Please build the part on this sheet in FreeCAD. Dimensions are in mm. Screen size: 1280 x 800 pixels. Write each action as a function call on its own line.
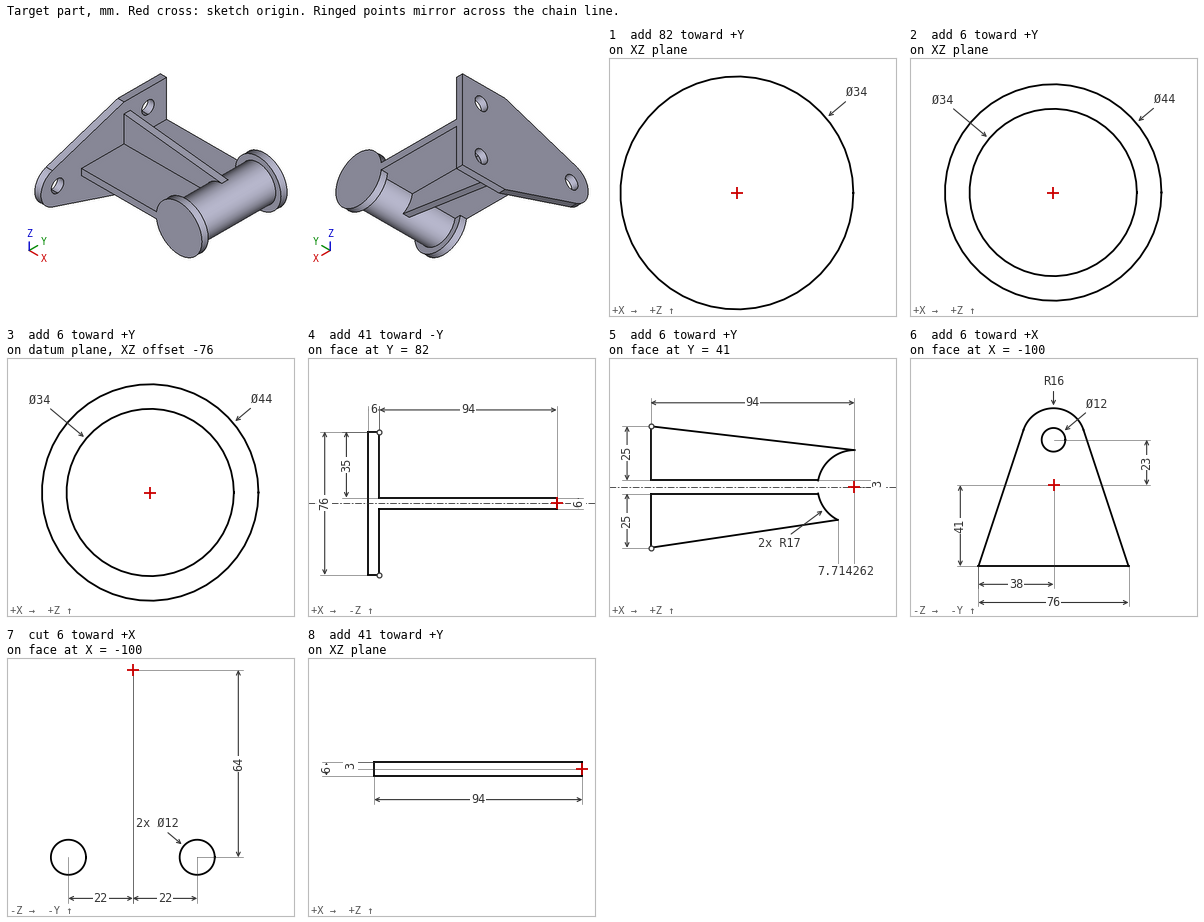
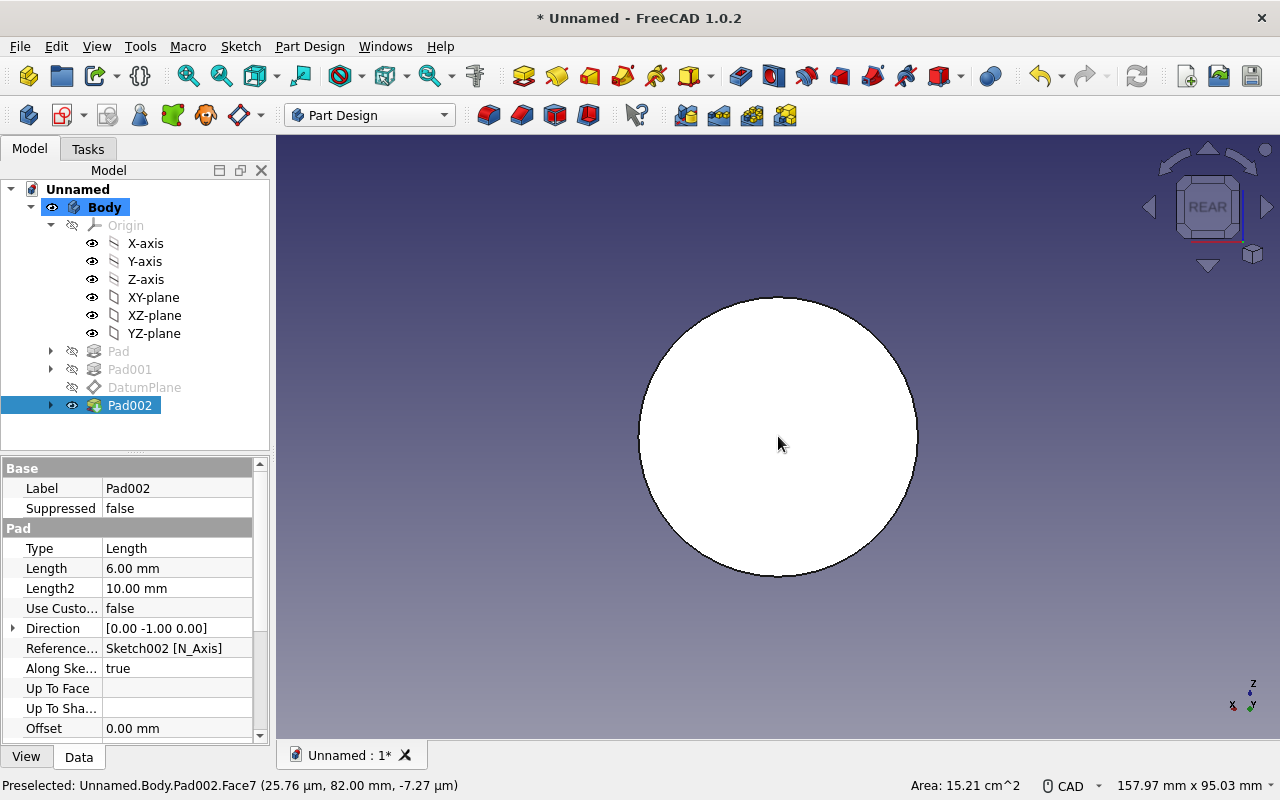
click(62, 116)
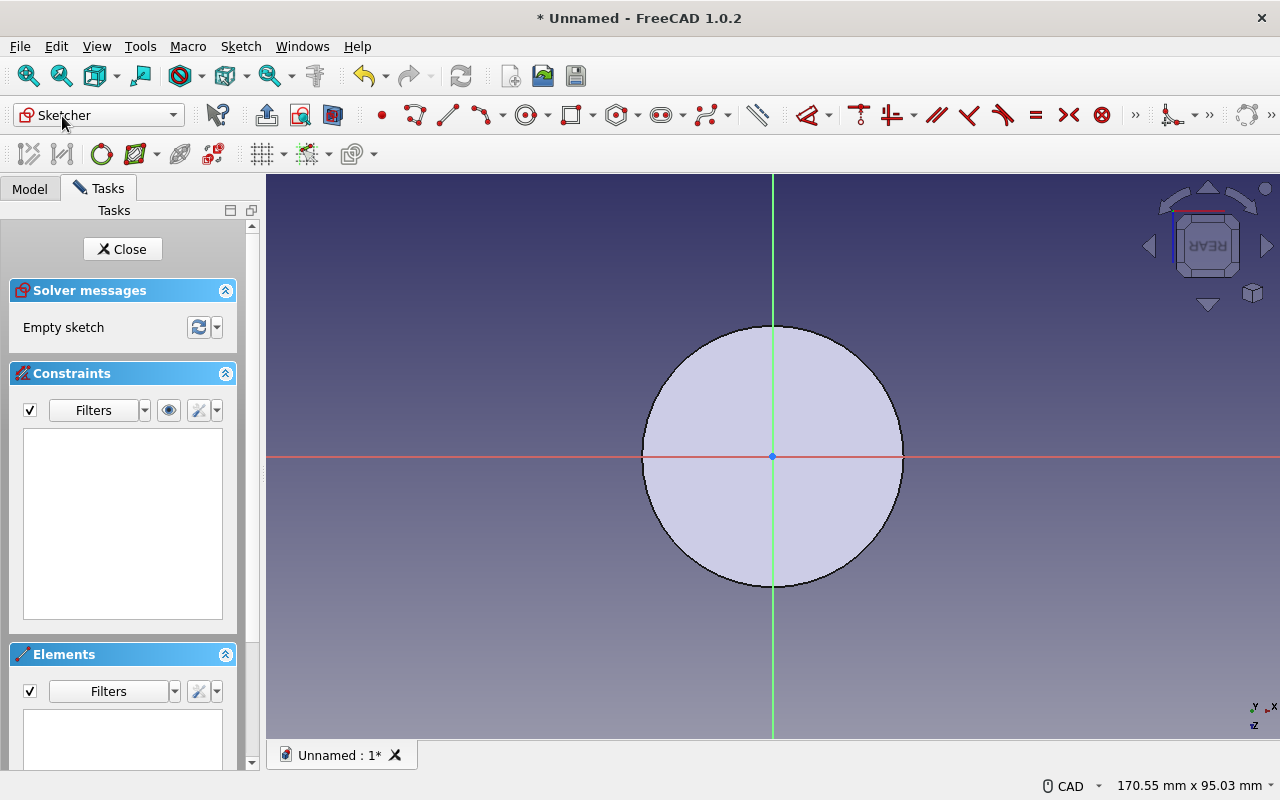
scroll(1115, 456, down, 1)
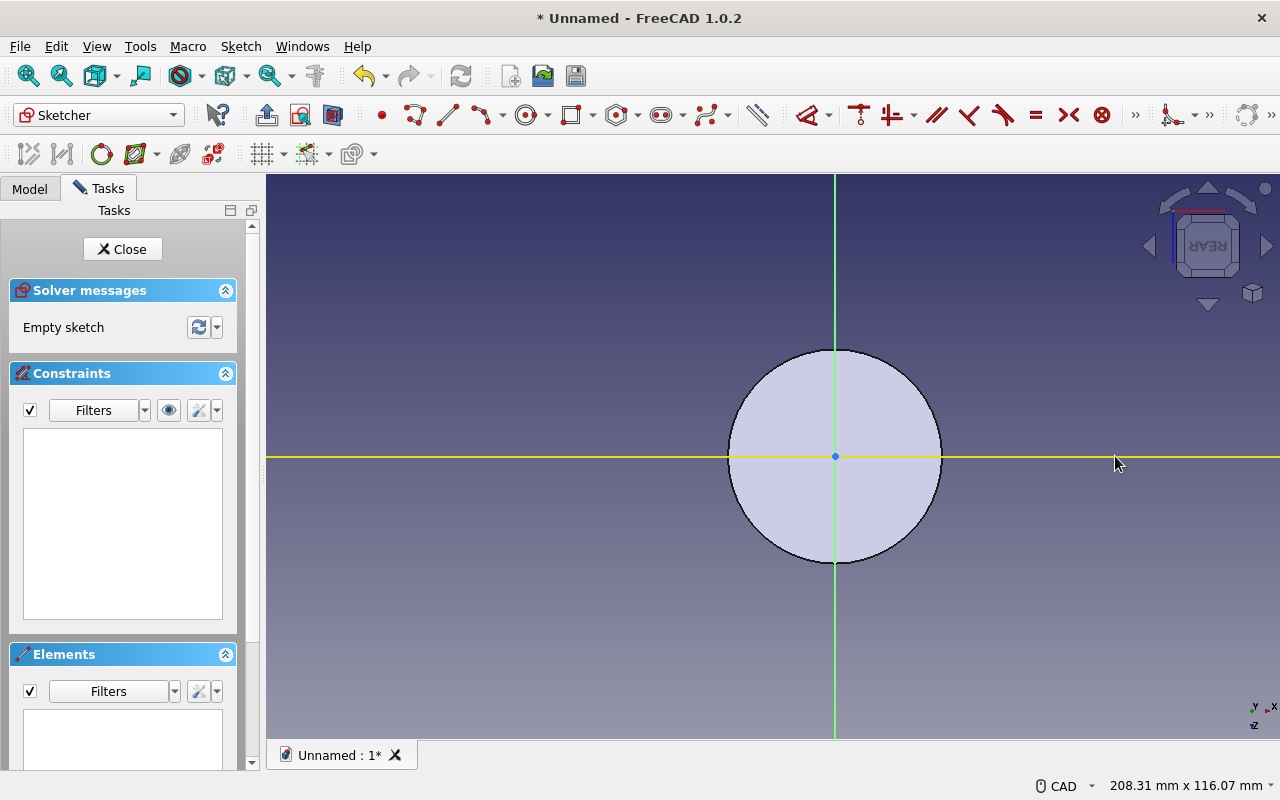
key(g)
key(m)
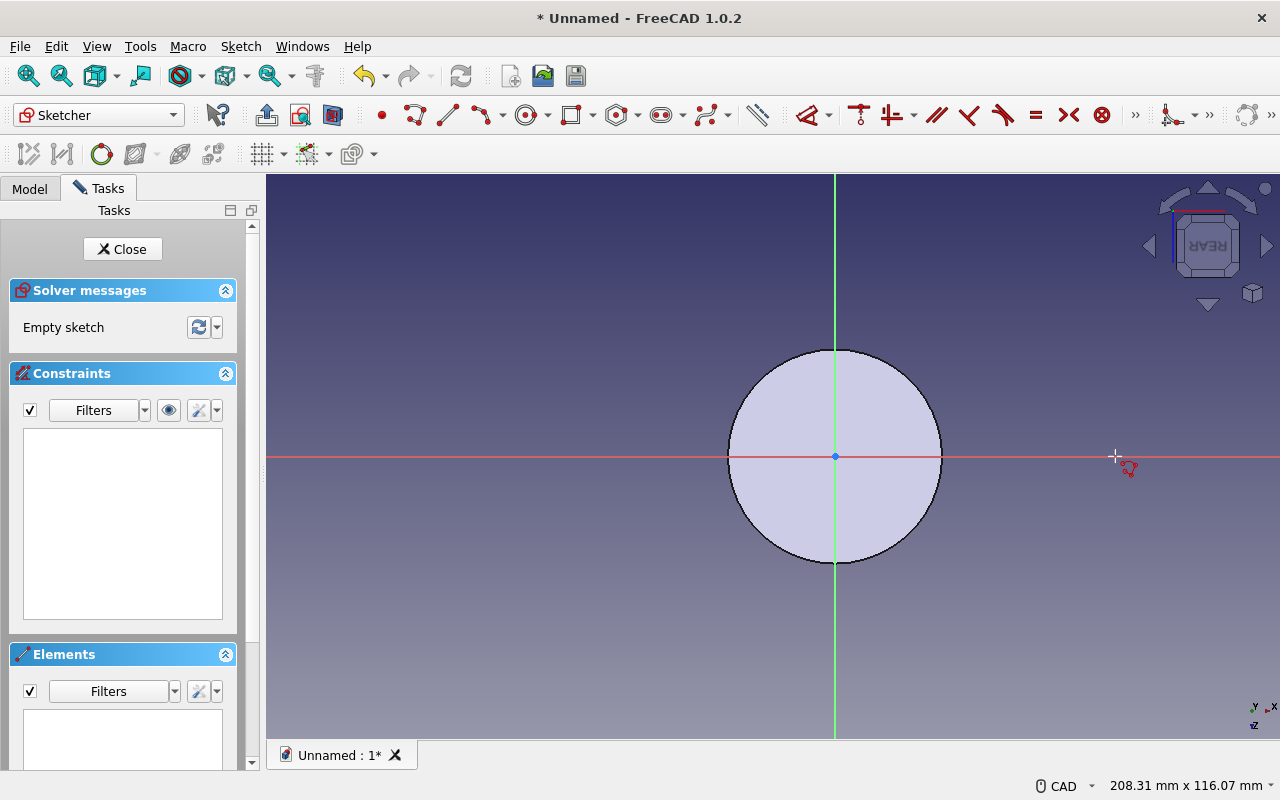
click(835, 471)
click(826, 442)
click(377, 442)
click(377, 272)
click(348, 272)
click(348, 642)
click(377, 642)
click(377, 471)
click(835, 472)
key(Escape)
key(Escape)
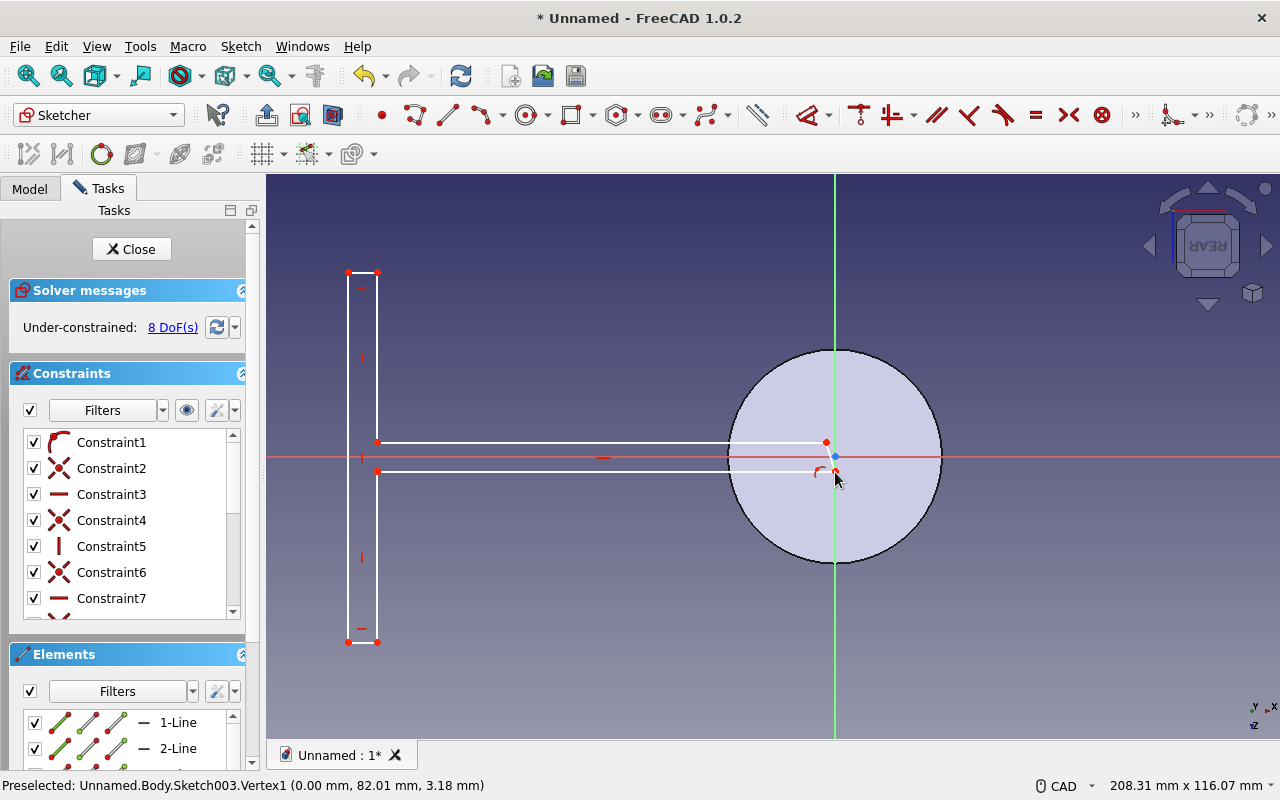
click(831, 460)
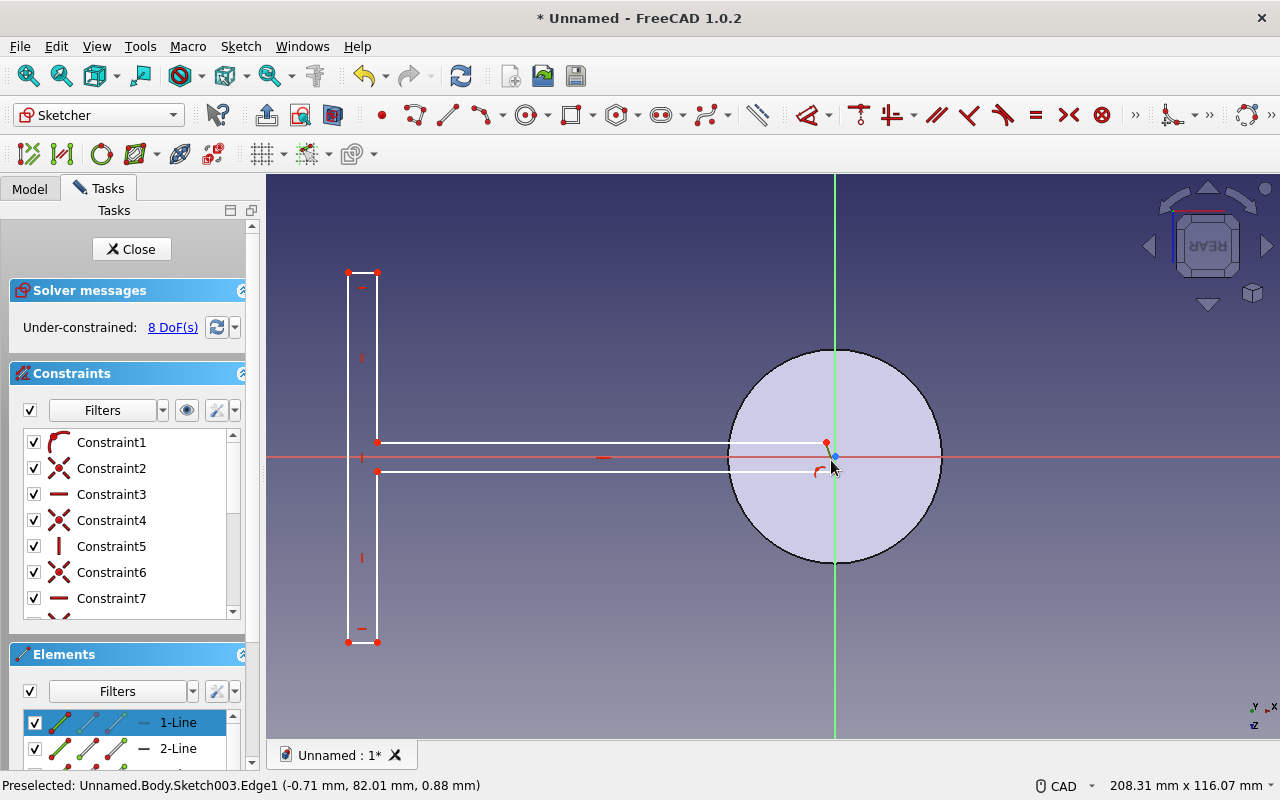
key(v)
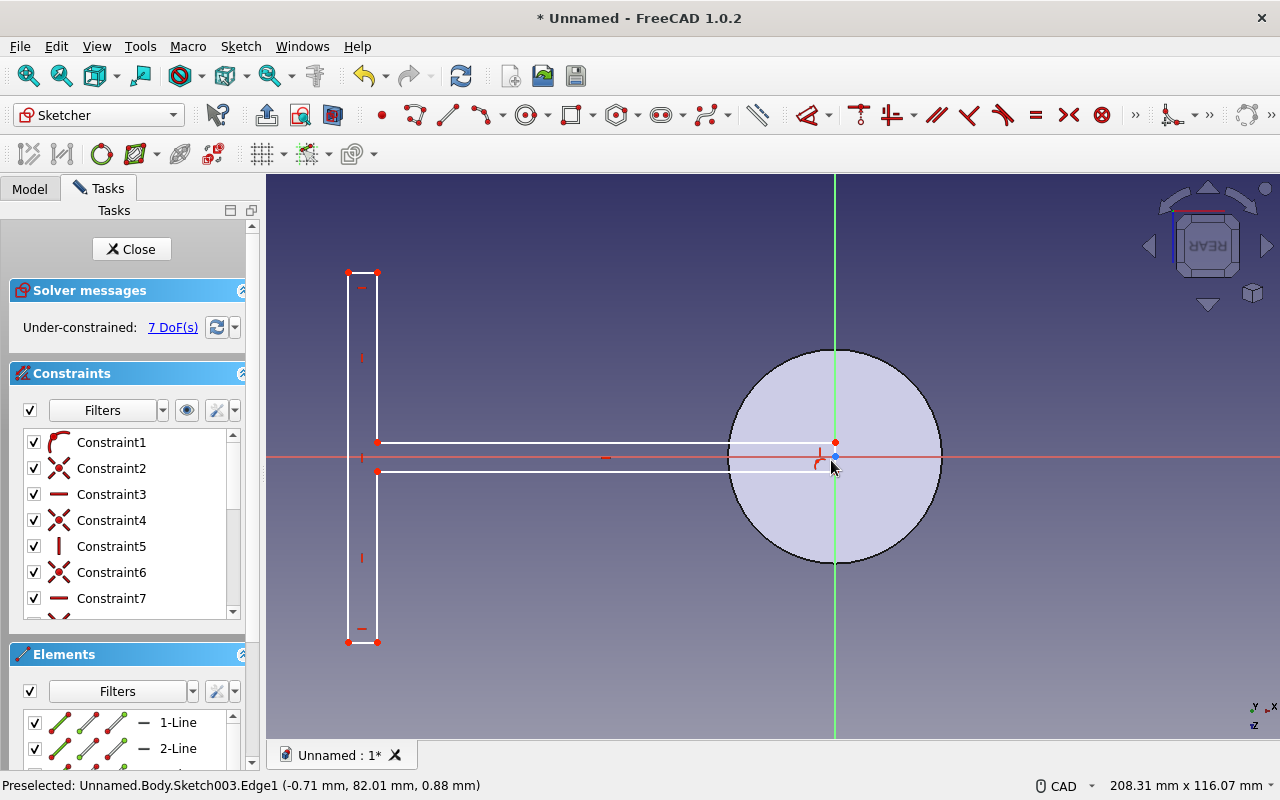
click(377, 273)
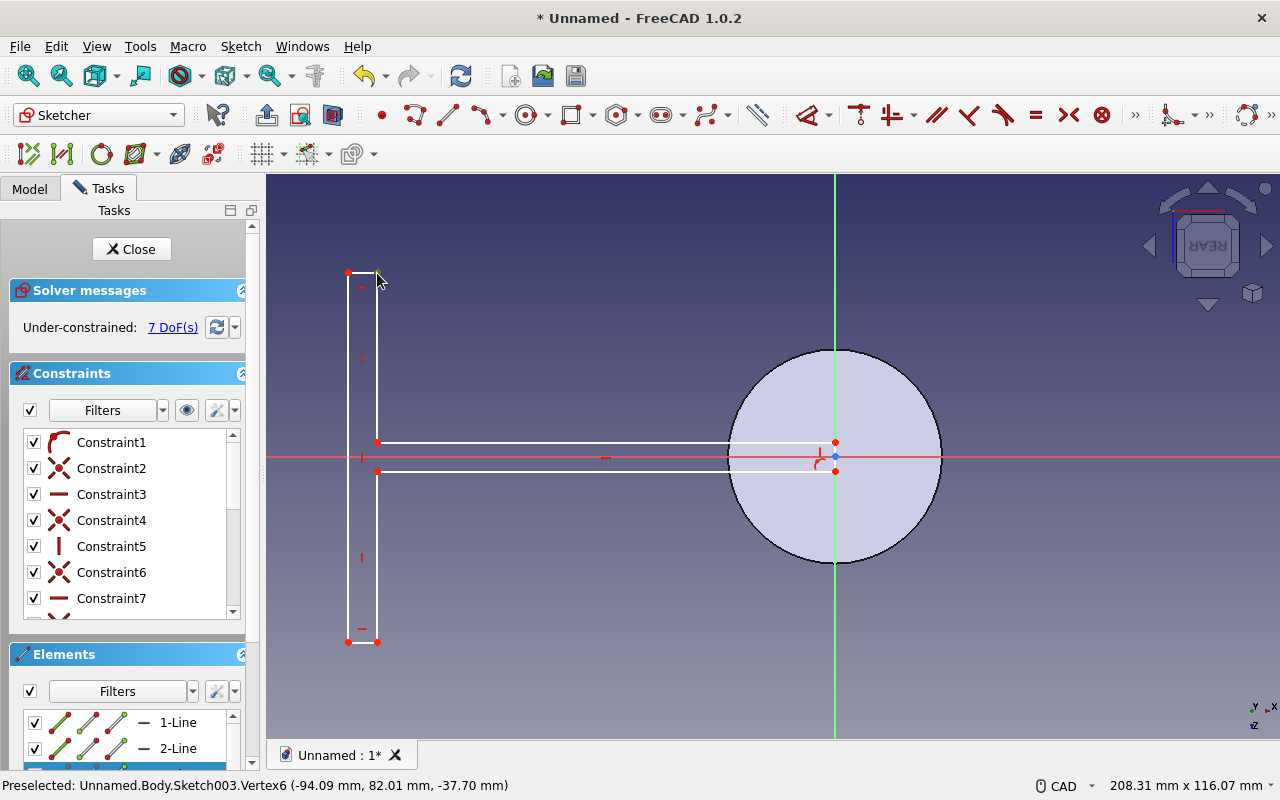
click(377, 643)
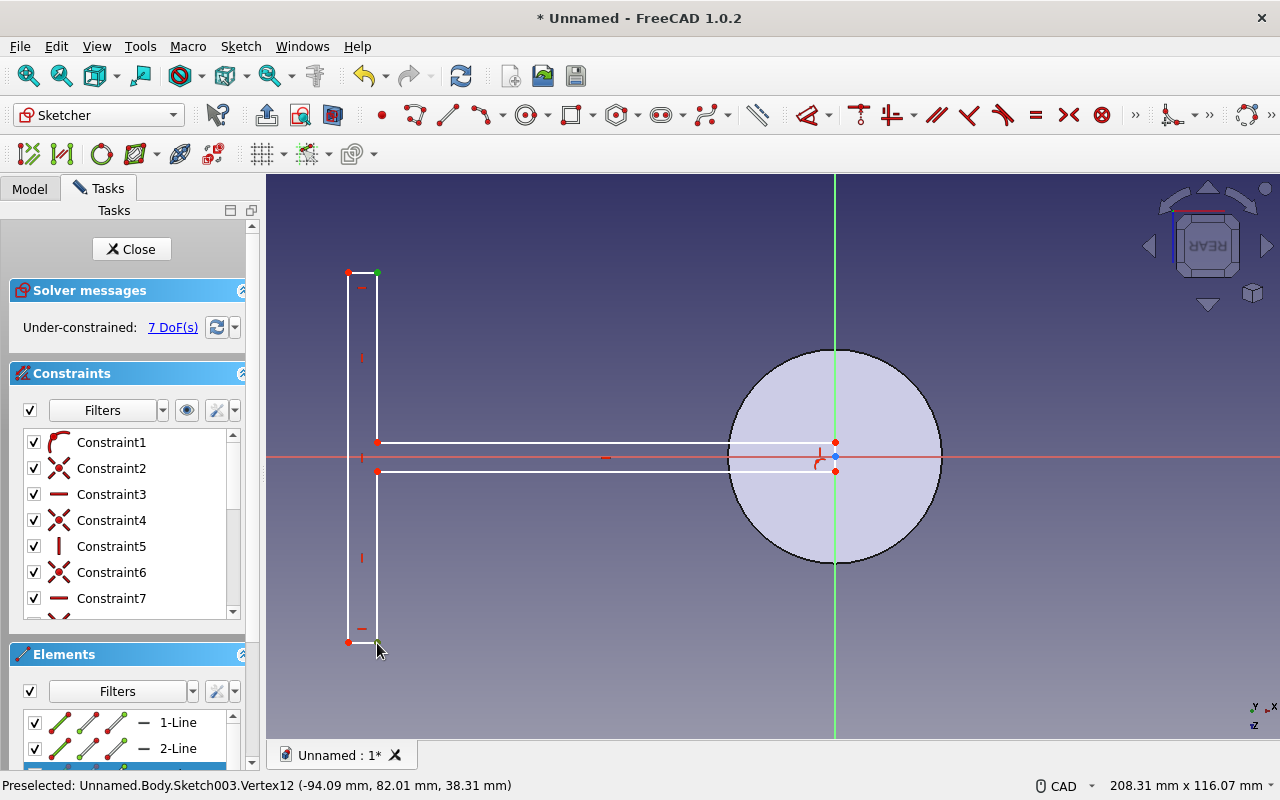
click(880, 457)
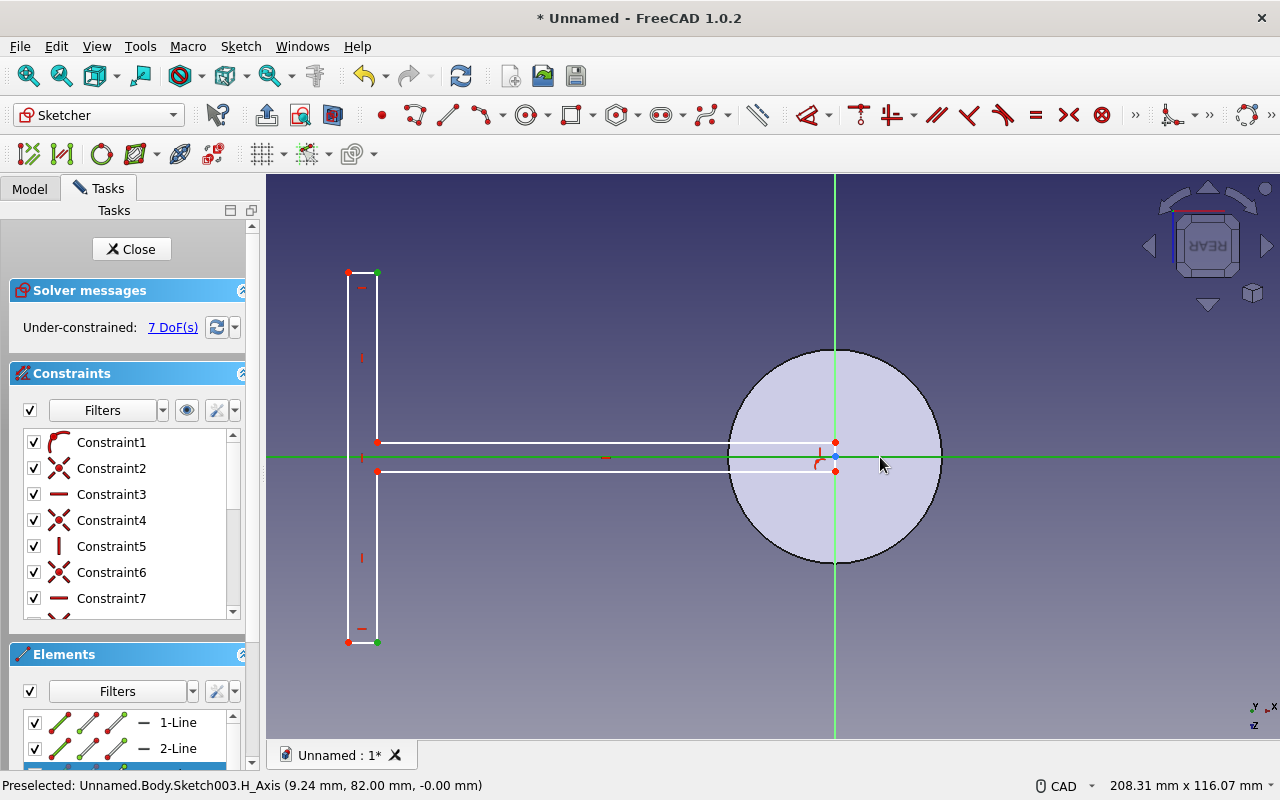
click(1069, 116)